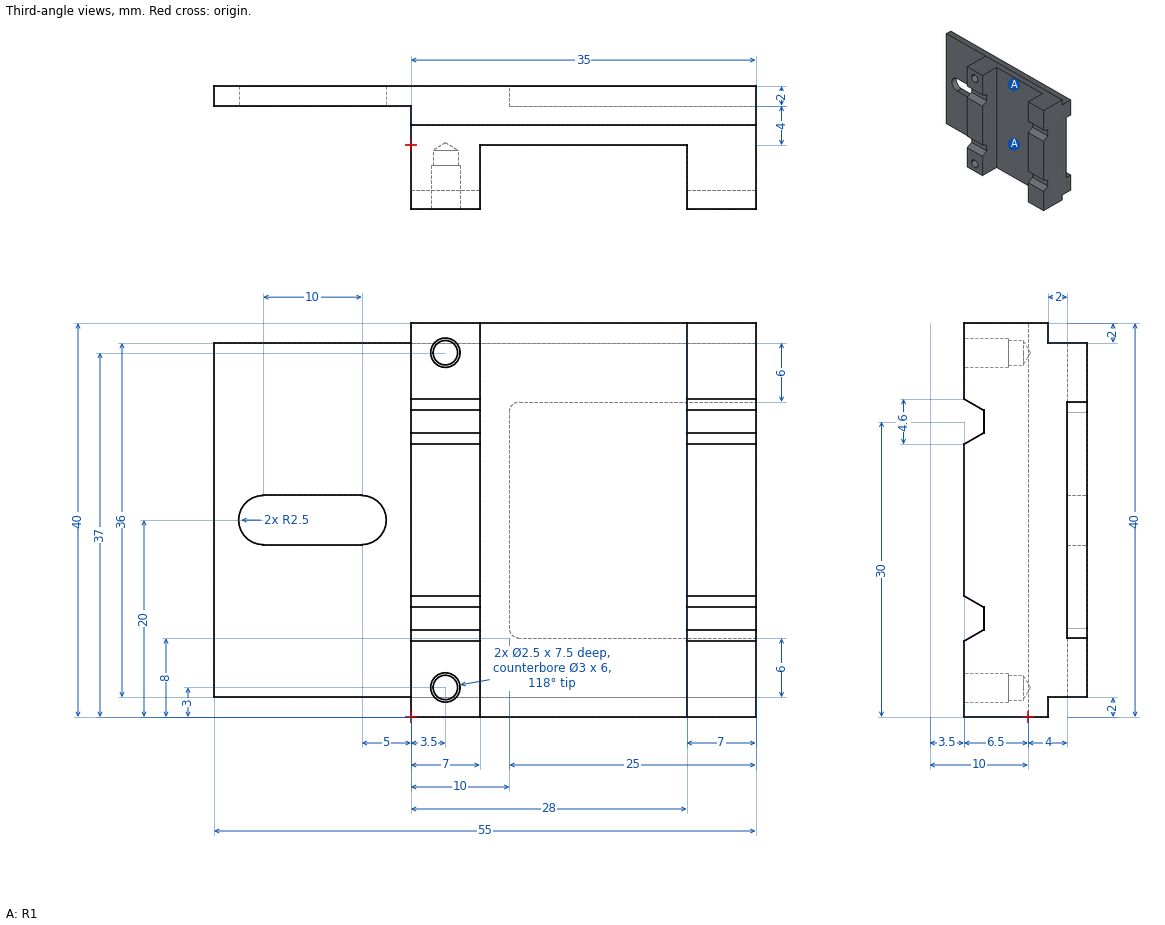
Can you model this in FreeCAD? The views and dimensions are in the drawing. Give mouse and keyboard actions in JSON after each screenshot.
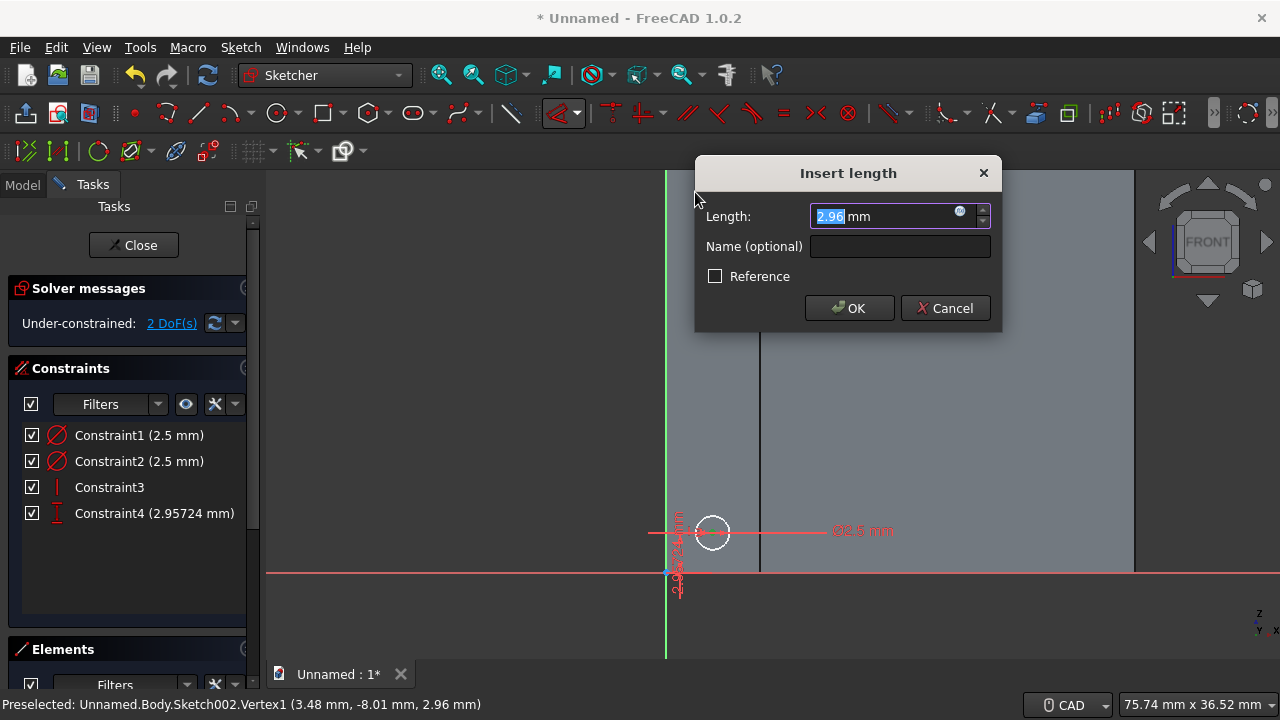
{"action": "type", "text": "3"}
{"action": "key", "text": "Return"}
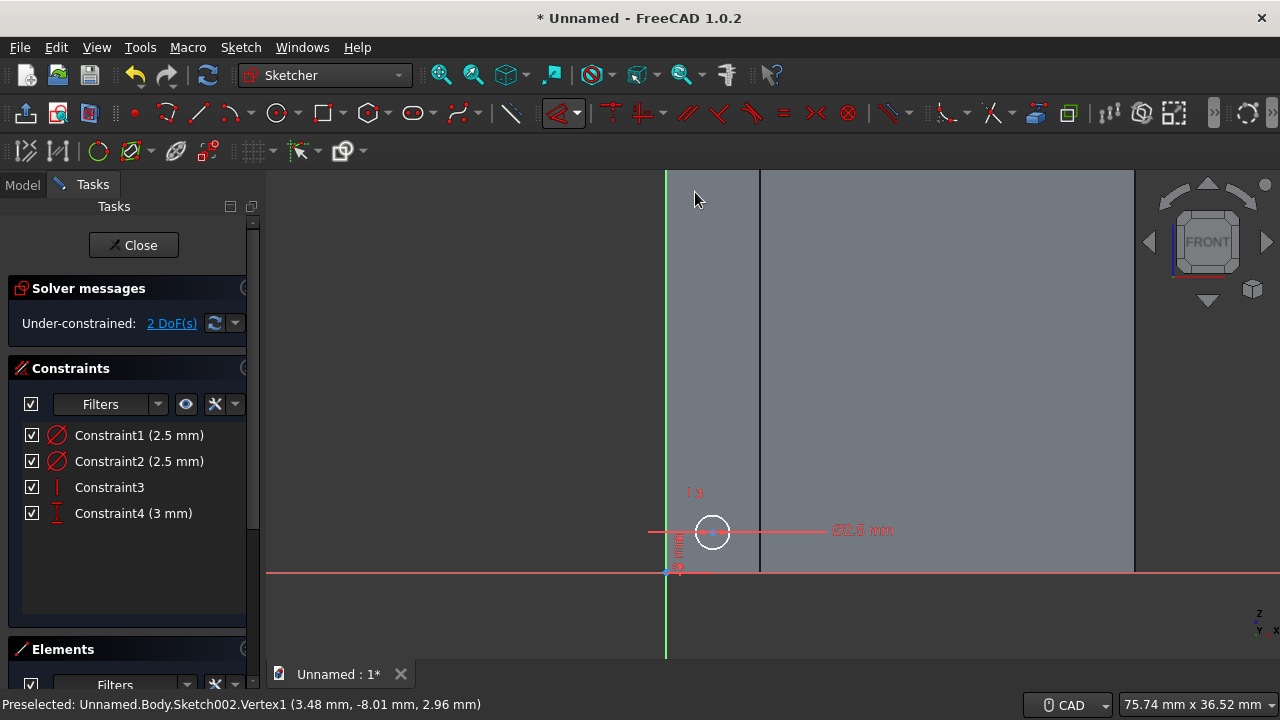
{"action": "scroll", "coordinate": [713, 534], "scroll_direction": "down", "scroll_amount": 3}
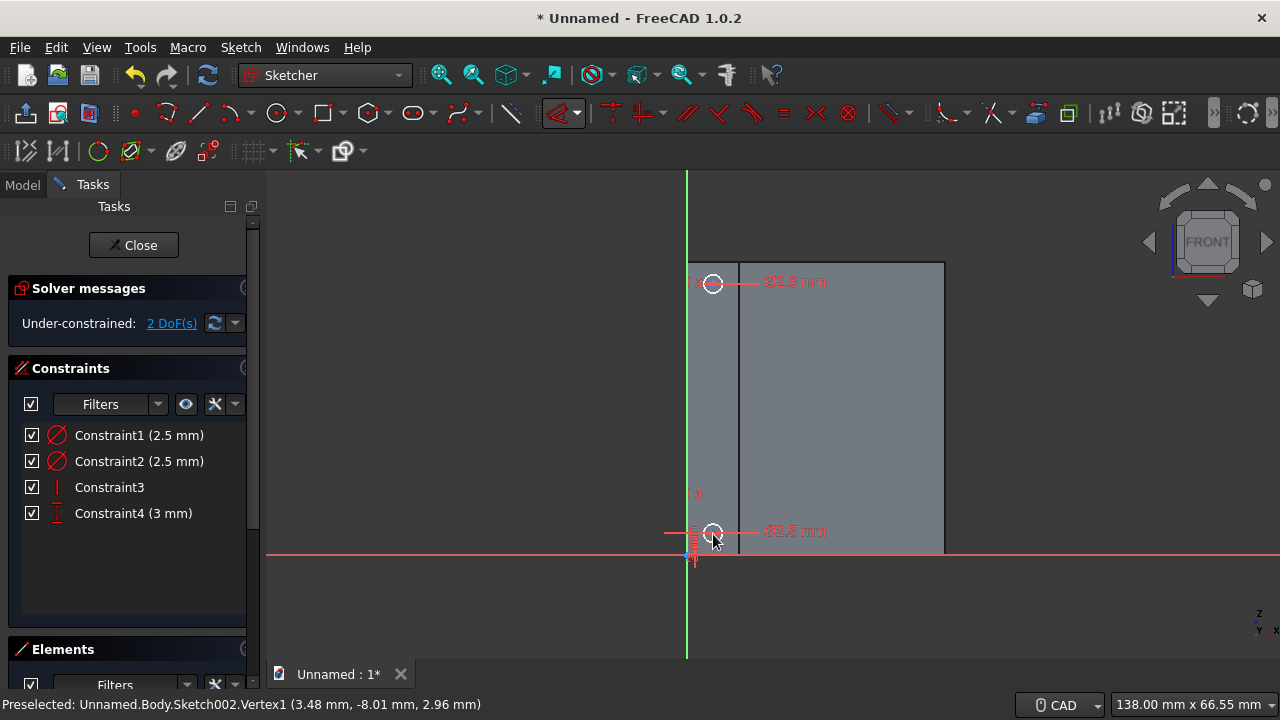
{"action": "left_click", "coordinate": [713, 284]}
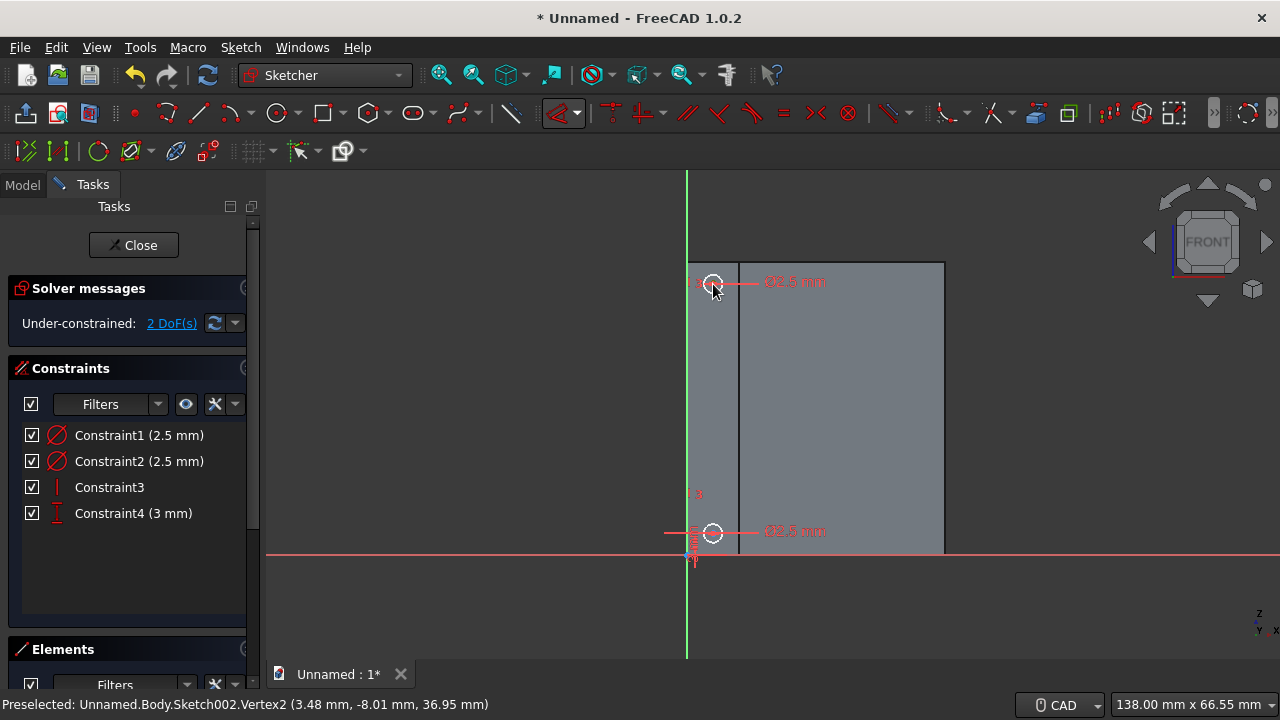
{"action": "key", "text": "i"}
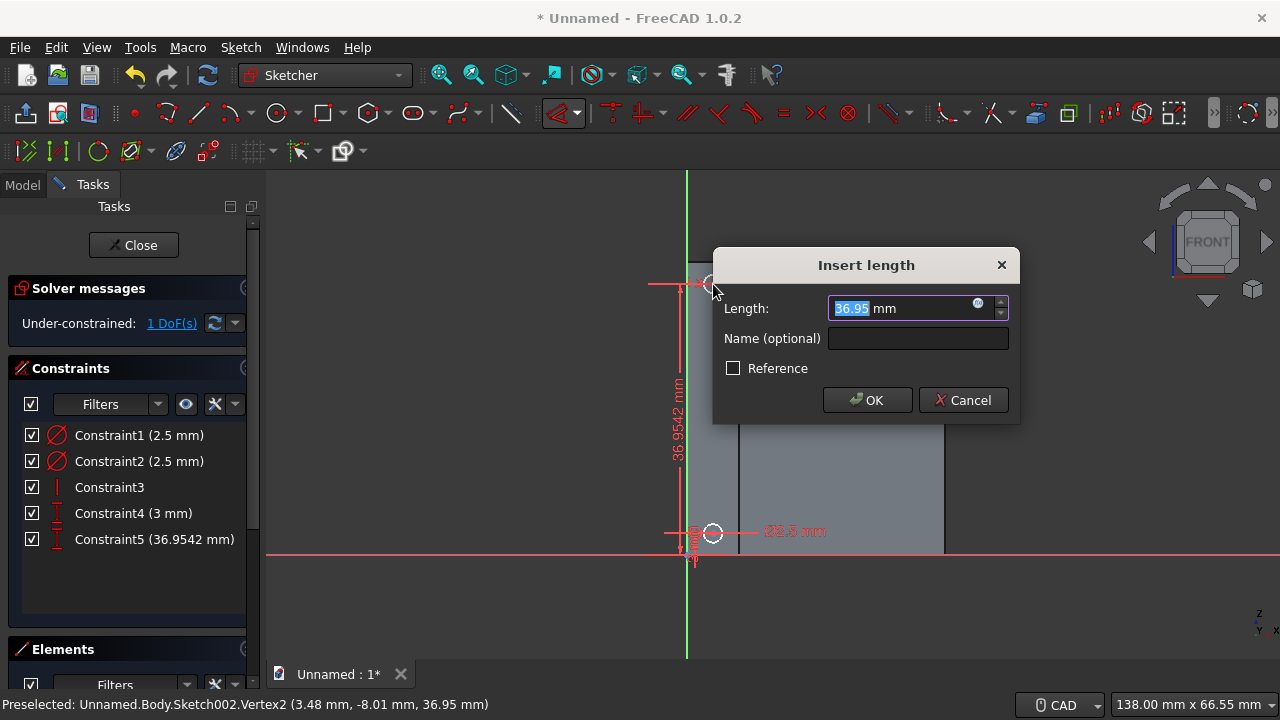
{"action": "type", "text": "37"}
{"action": "key", "text": "Return"}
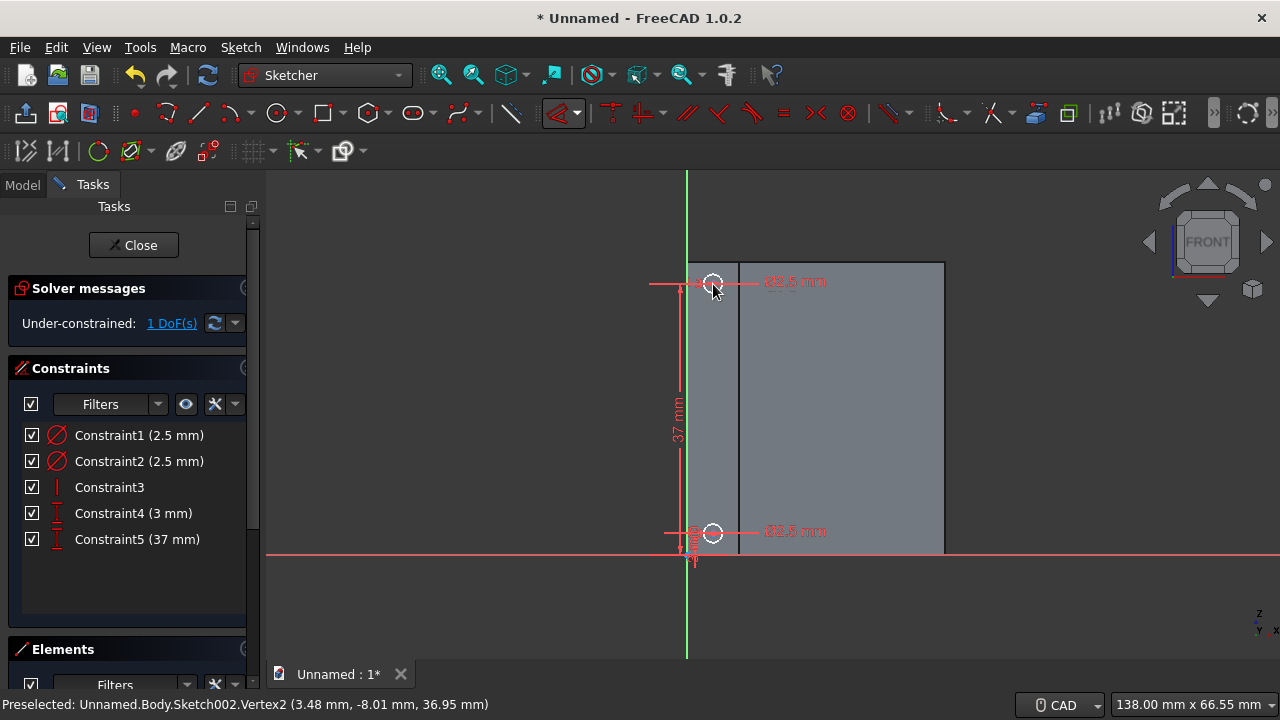
{"action": "scroll", "coordinate": [713, 533], "scroll_direction": "up", "scroll_amount": 3}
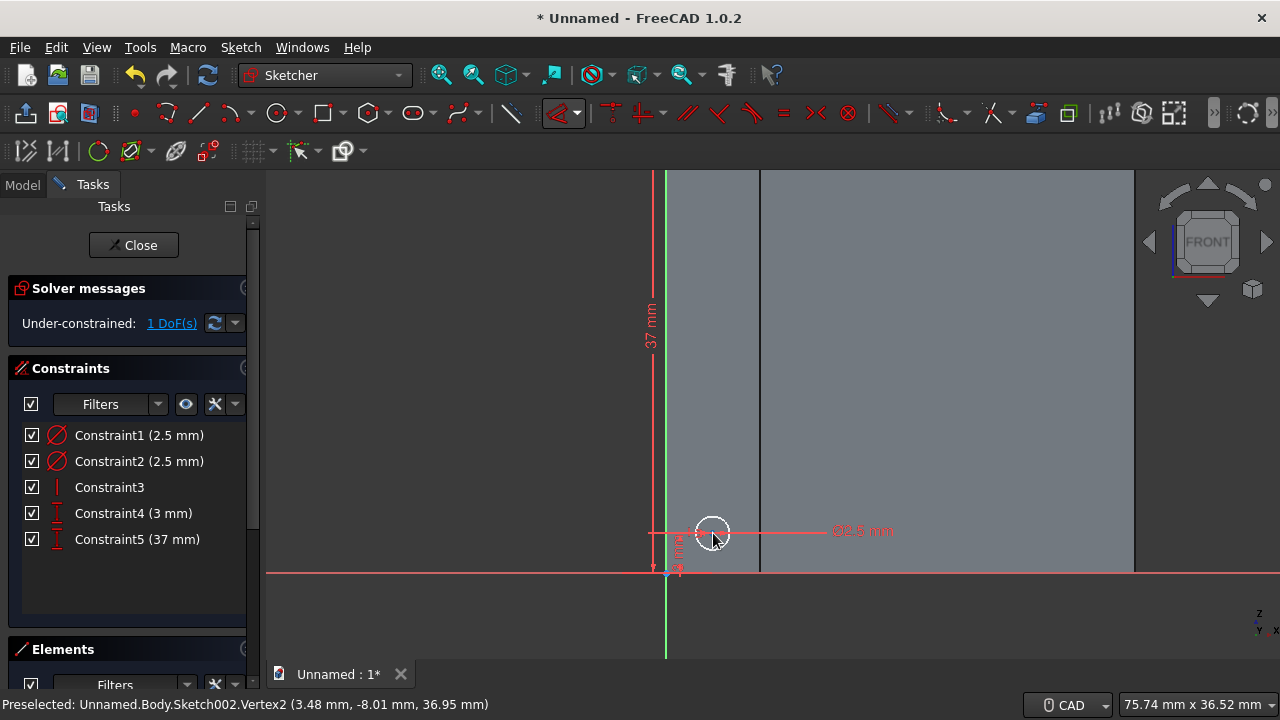
{"action": "left_click", "coordinate": [713, 533]}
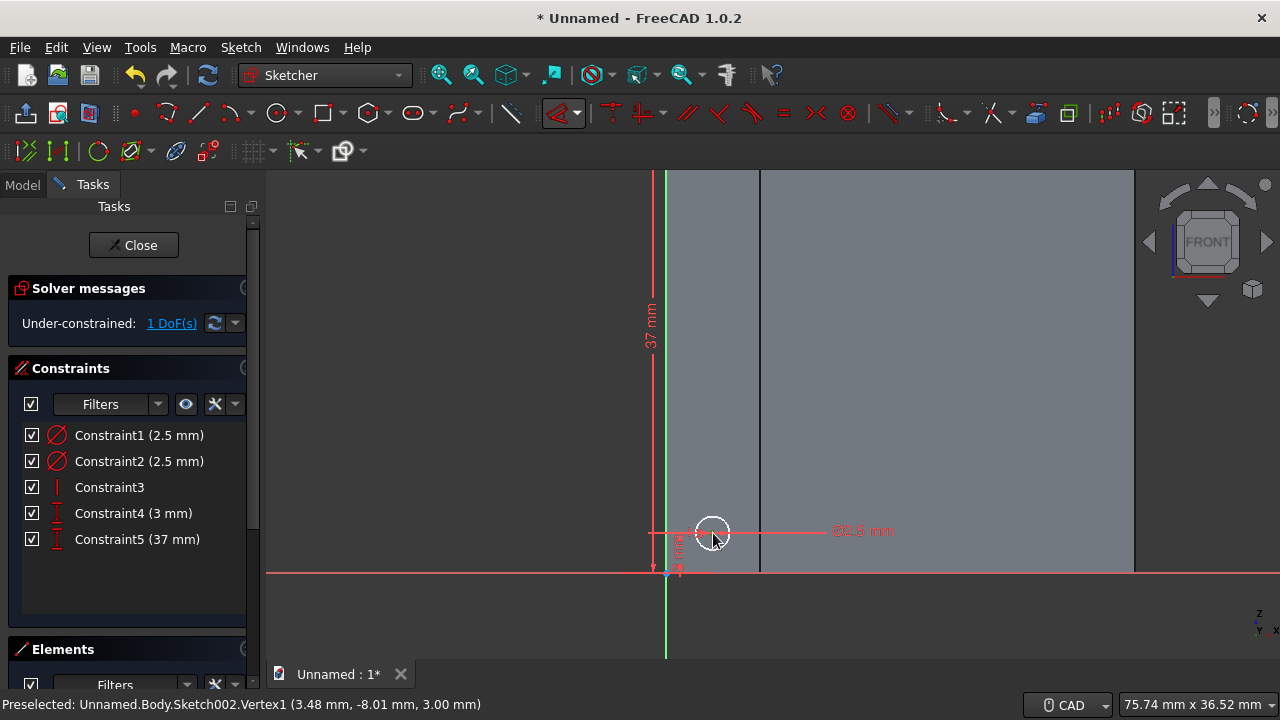
{"action": "left_click", "coordinate": [580, 114]}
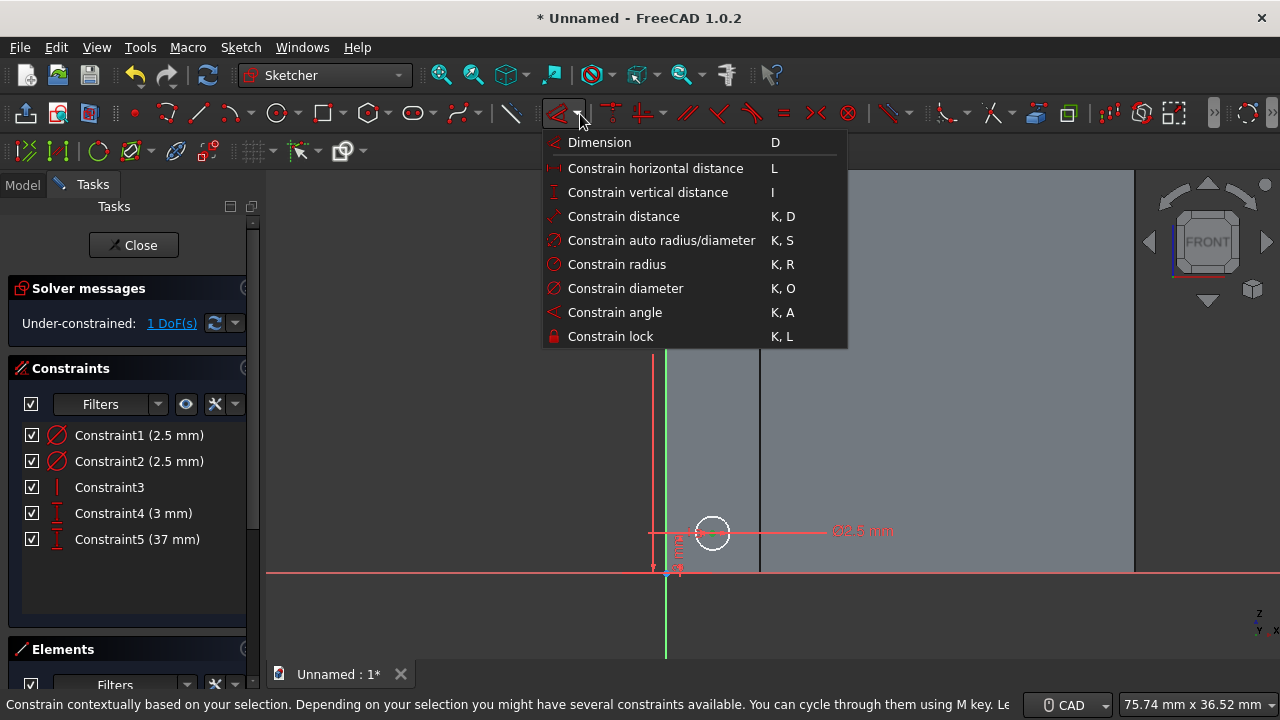
{"action": "left_click", "coordinate": [695, 168]}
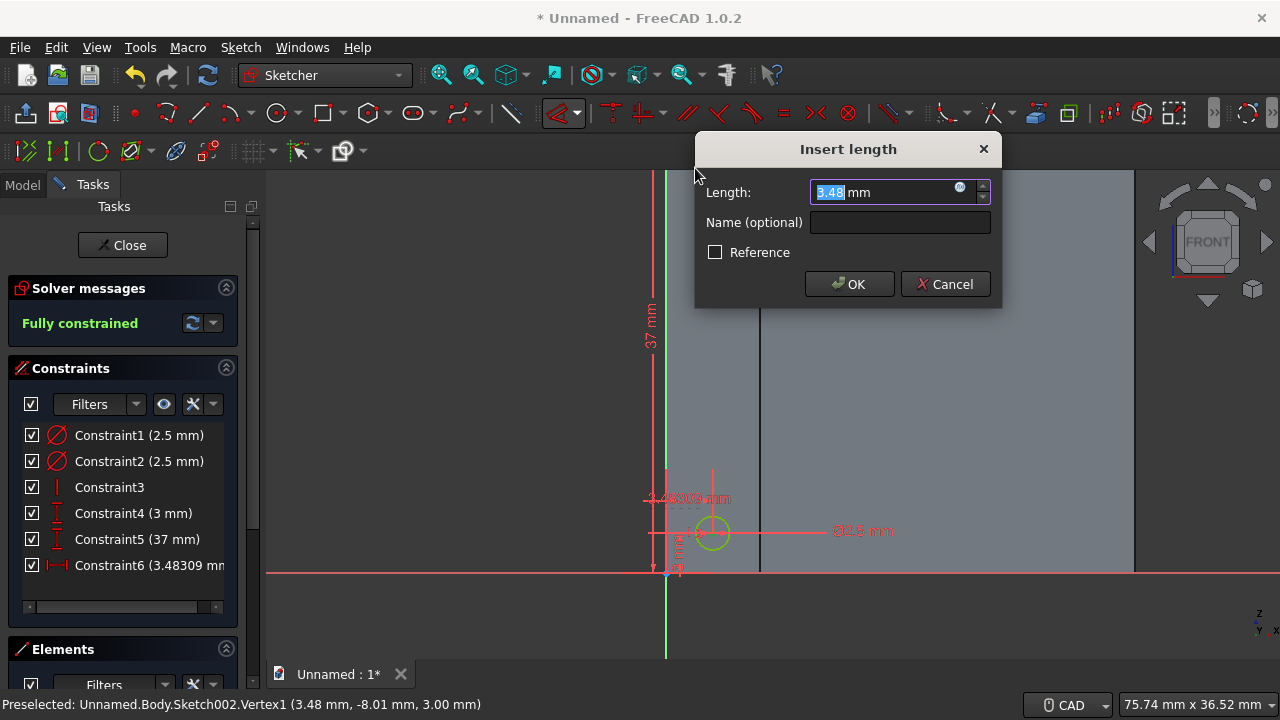
{"action": "type", "text": "3.5"}
{"action": "key", "text": "Return"}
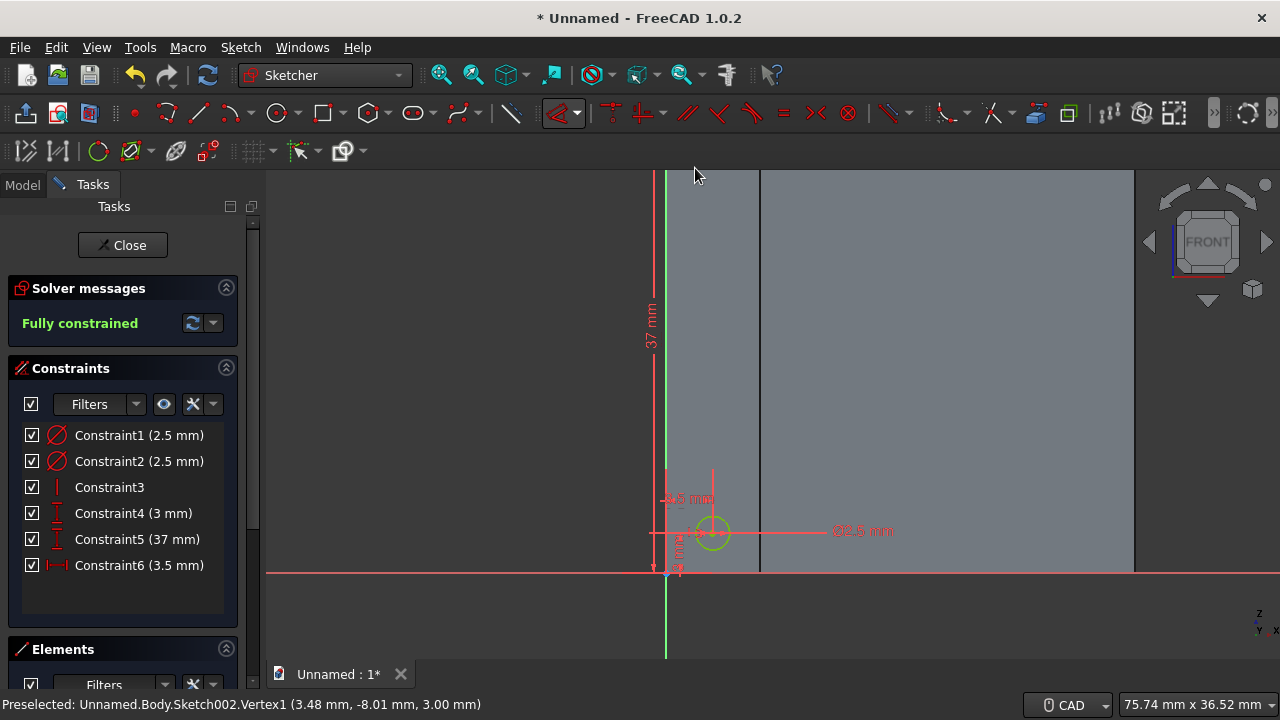
{"action": "left_click", "coordinate": [123, 245]}